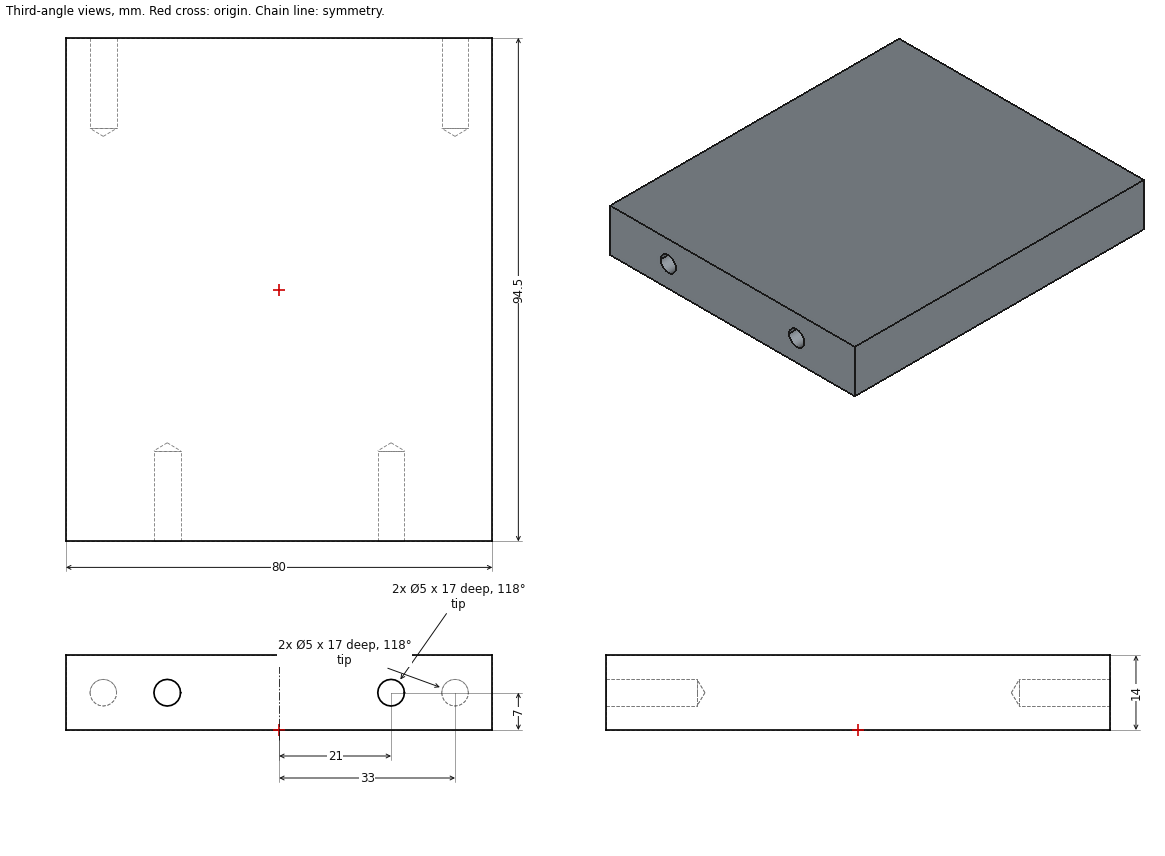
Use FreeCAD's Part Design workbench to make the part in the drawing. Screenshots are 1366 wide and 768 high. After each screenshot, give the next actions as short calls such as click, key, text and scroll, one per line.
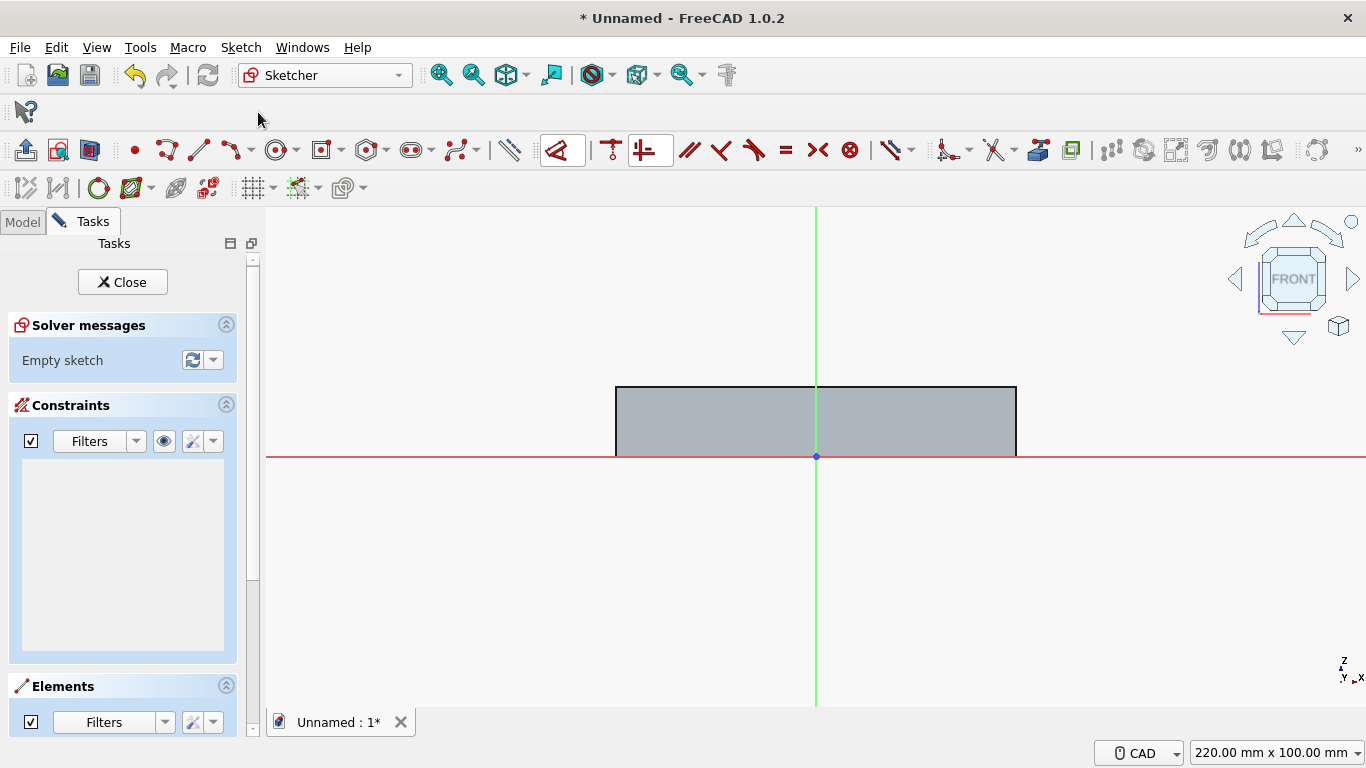
scroll(856, 419, up, 5)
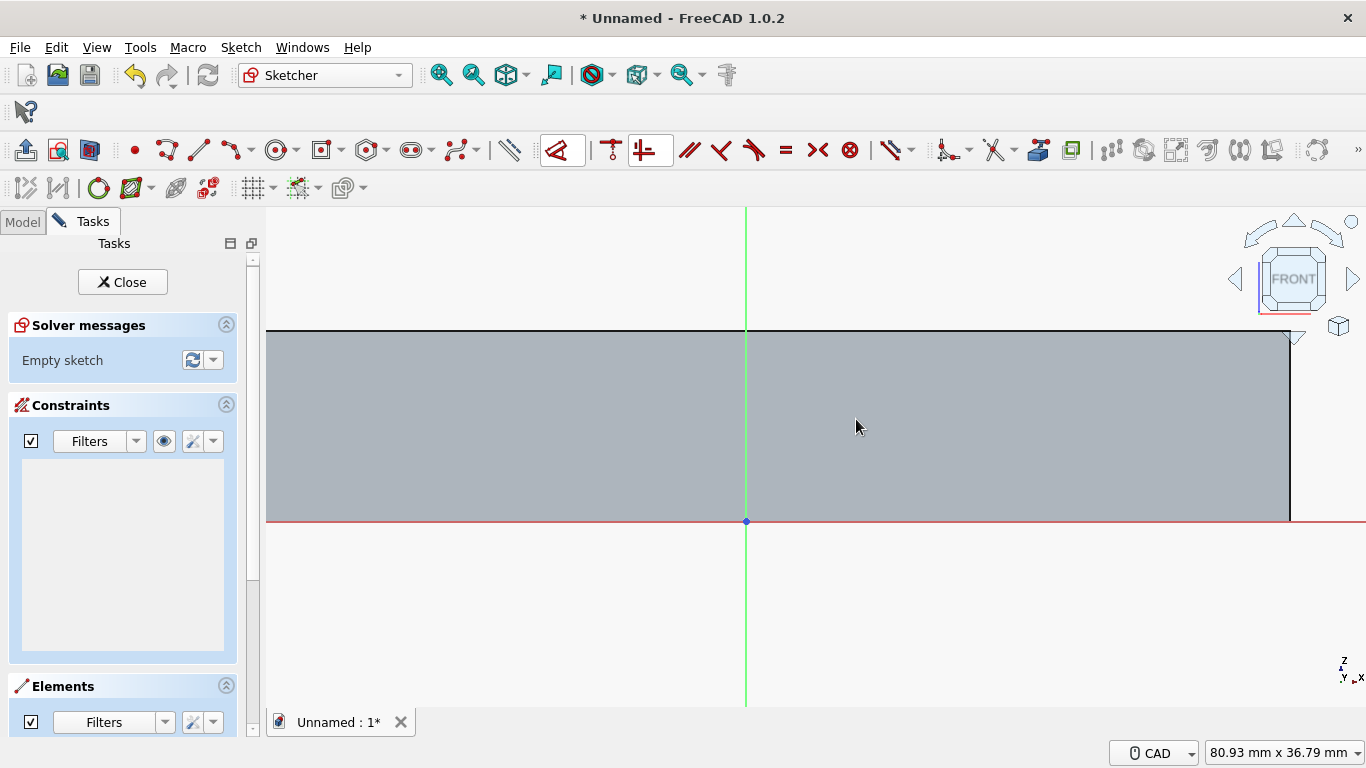
key(g)
key(c)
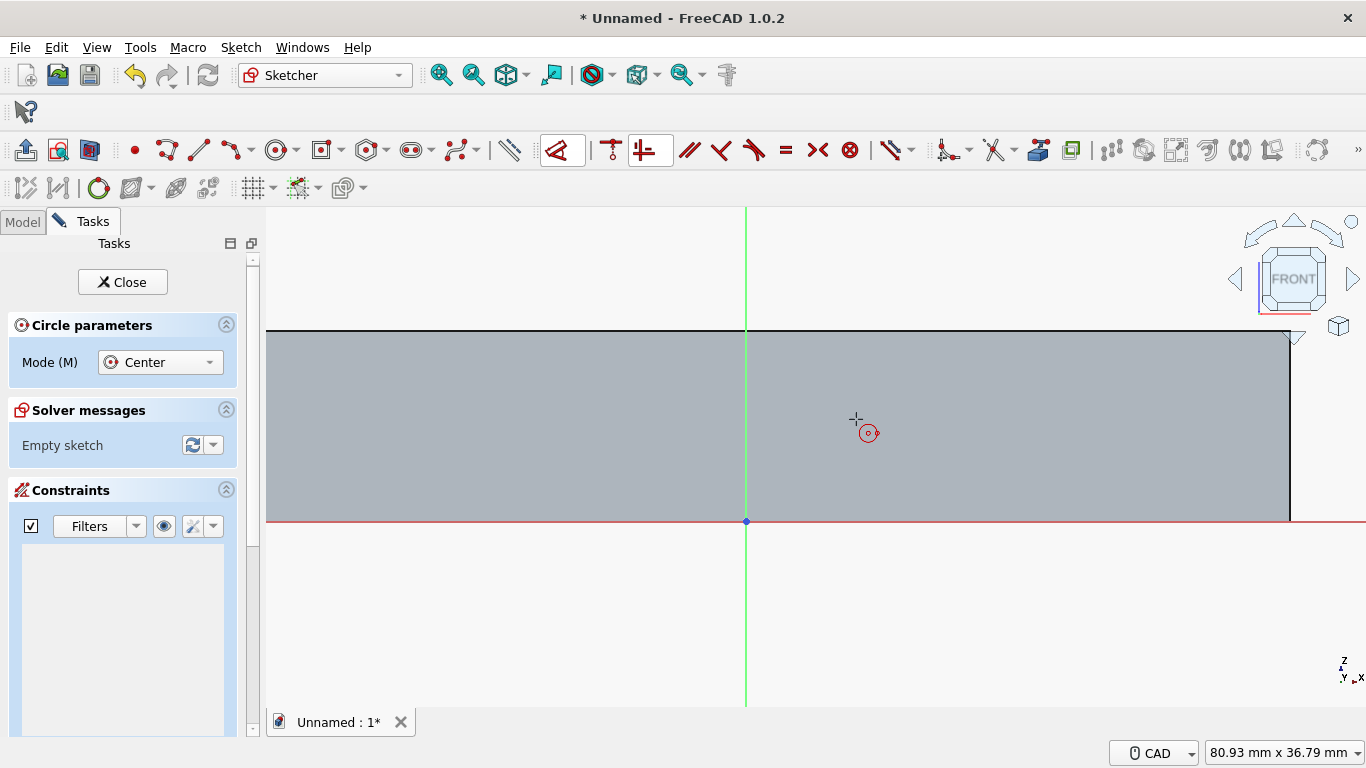
click(1032, 426)
click(1056, 402)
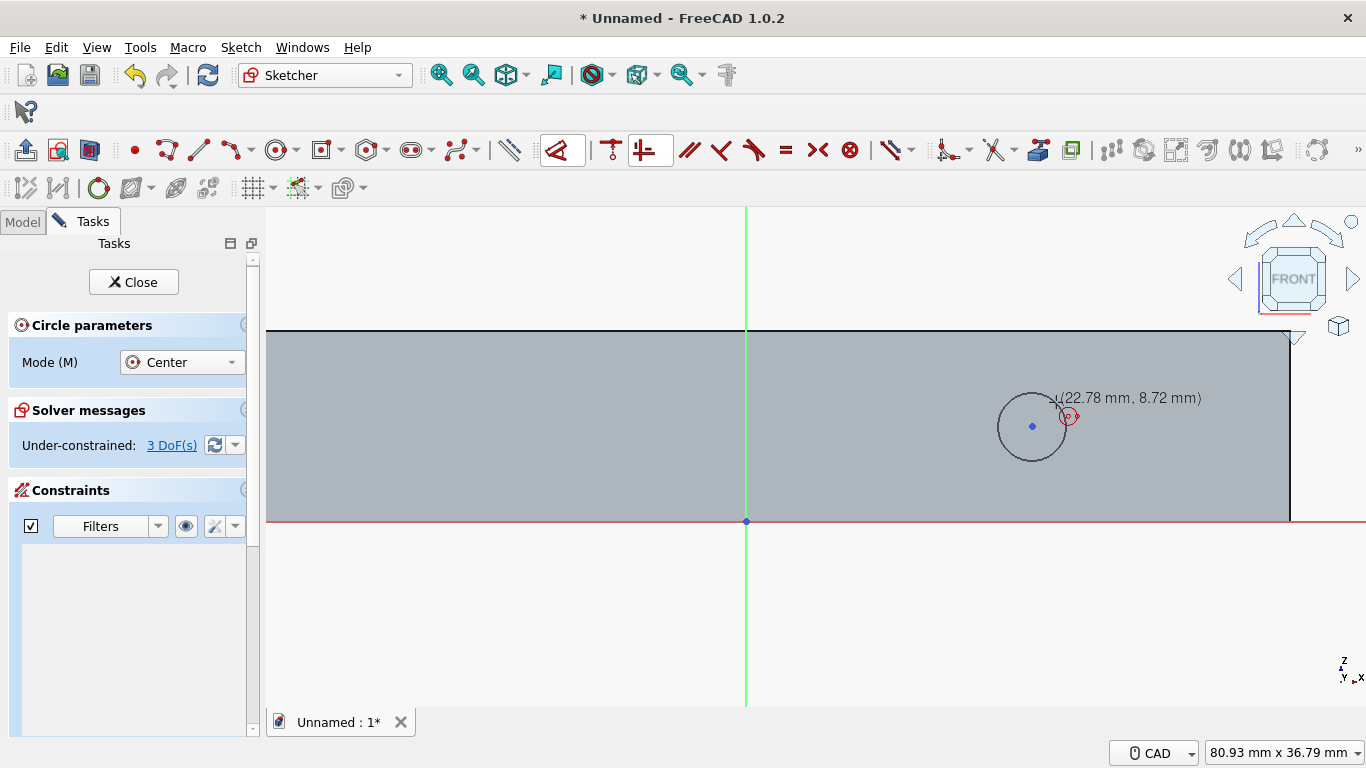
click(461, 426)
click(485, 402)
key(Escape)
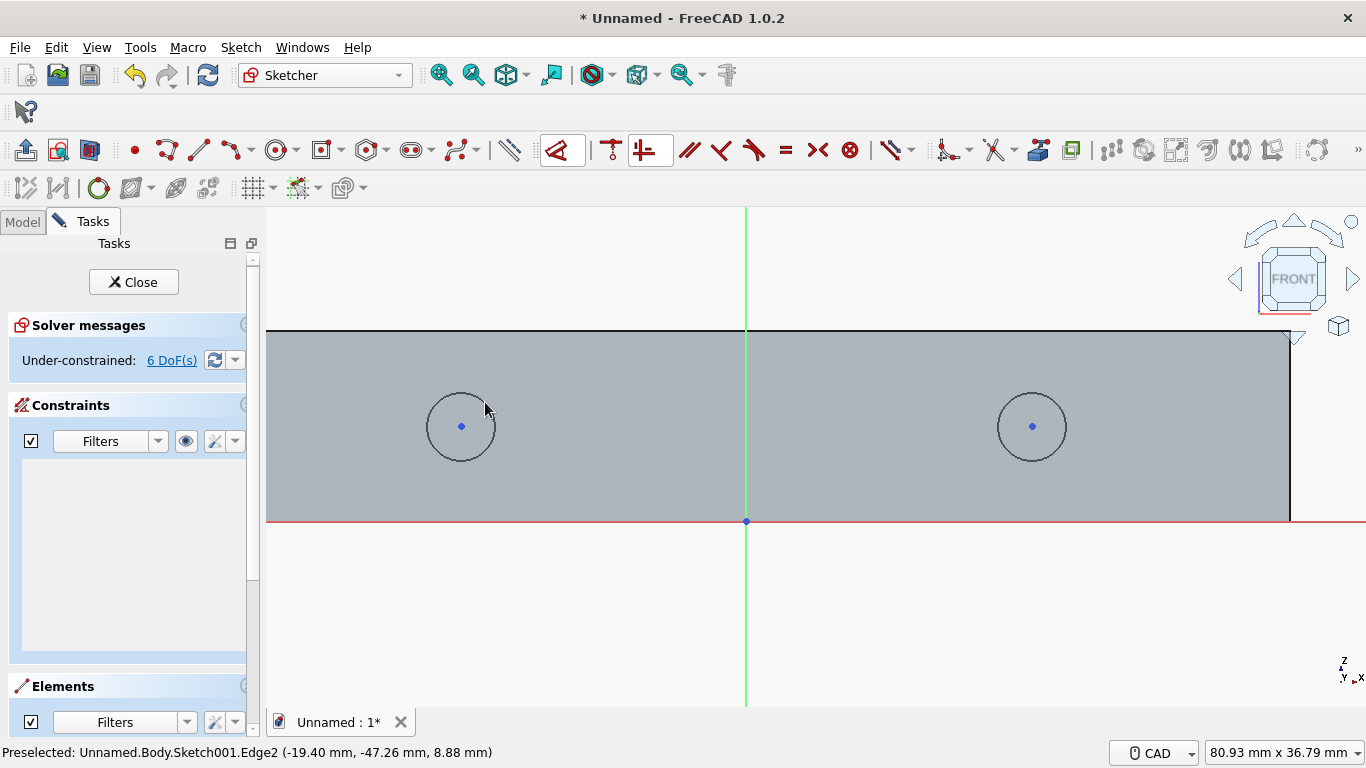
click(1056, 403)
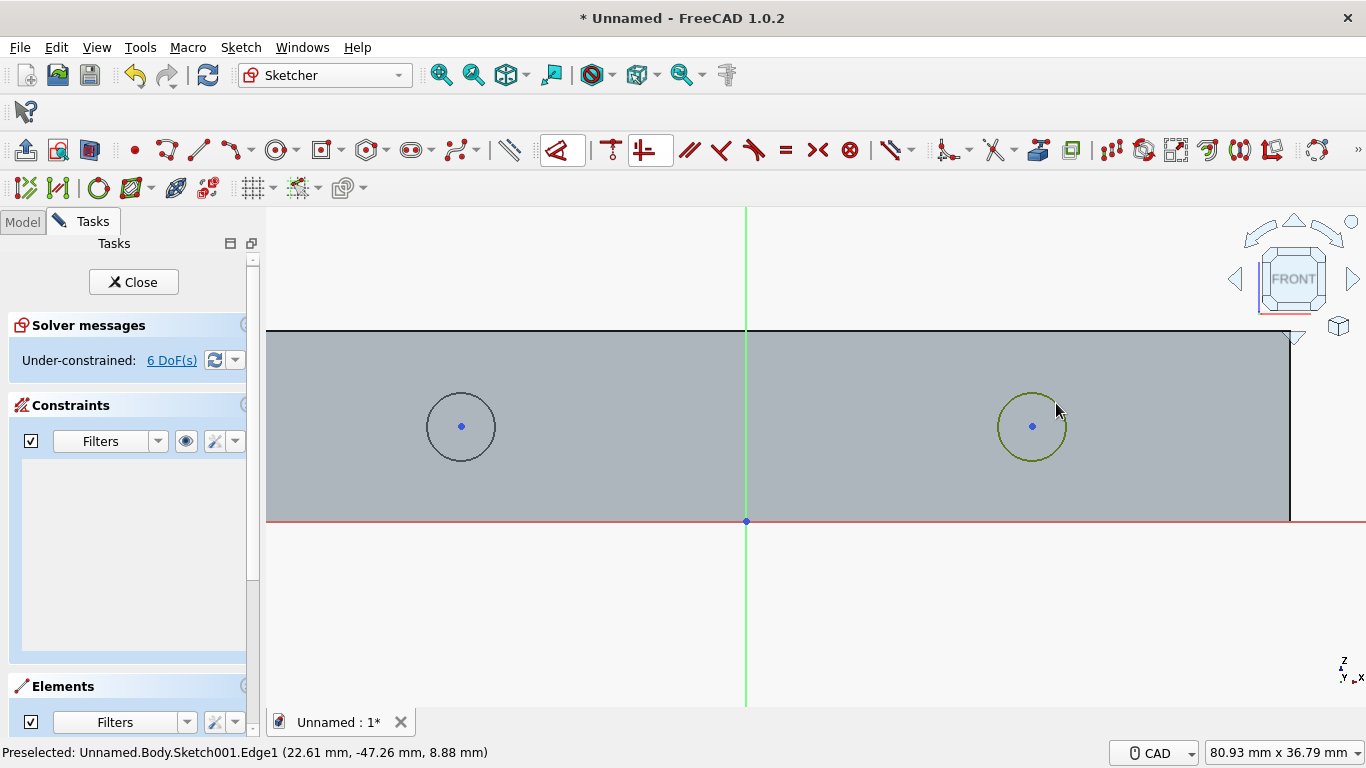
click(485, 403)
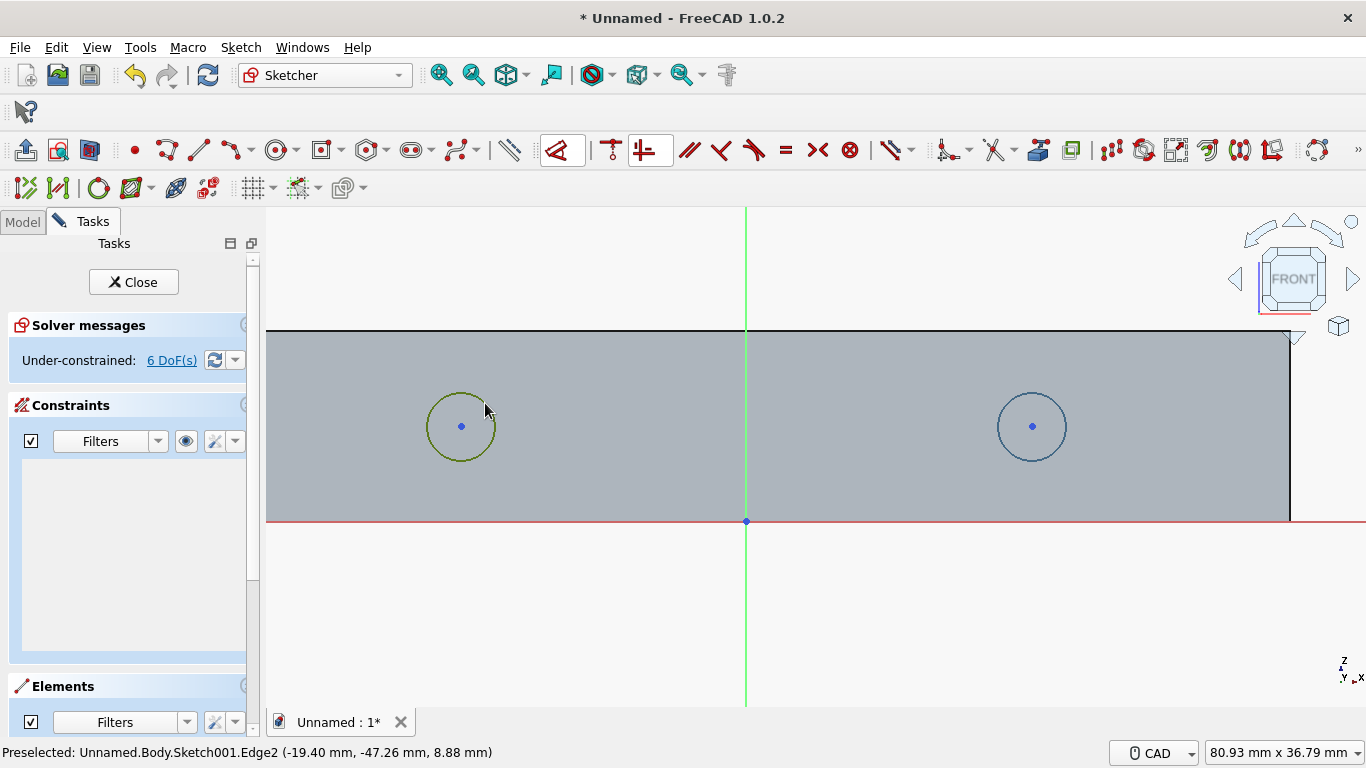
key(e)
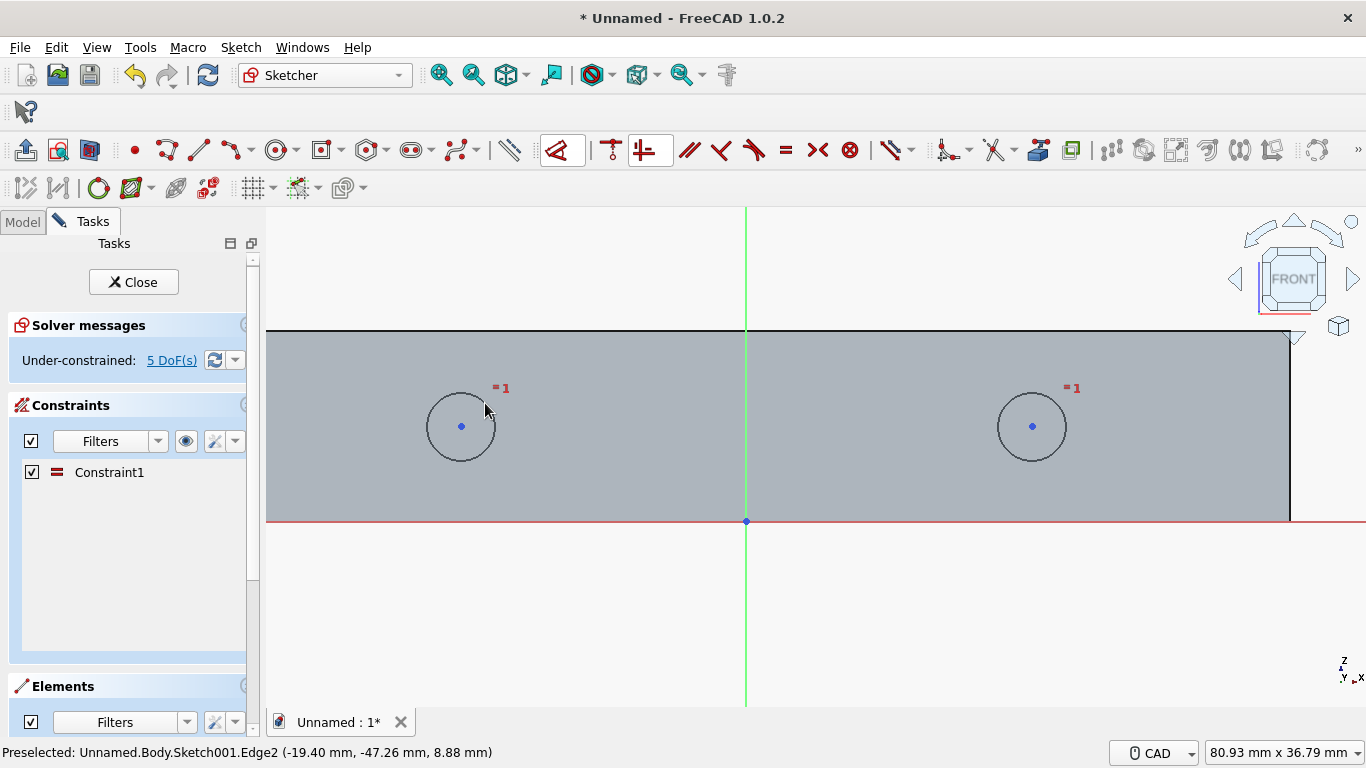
click(1032, 427)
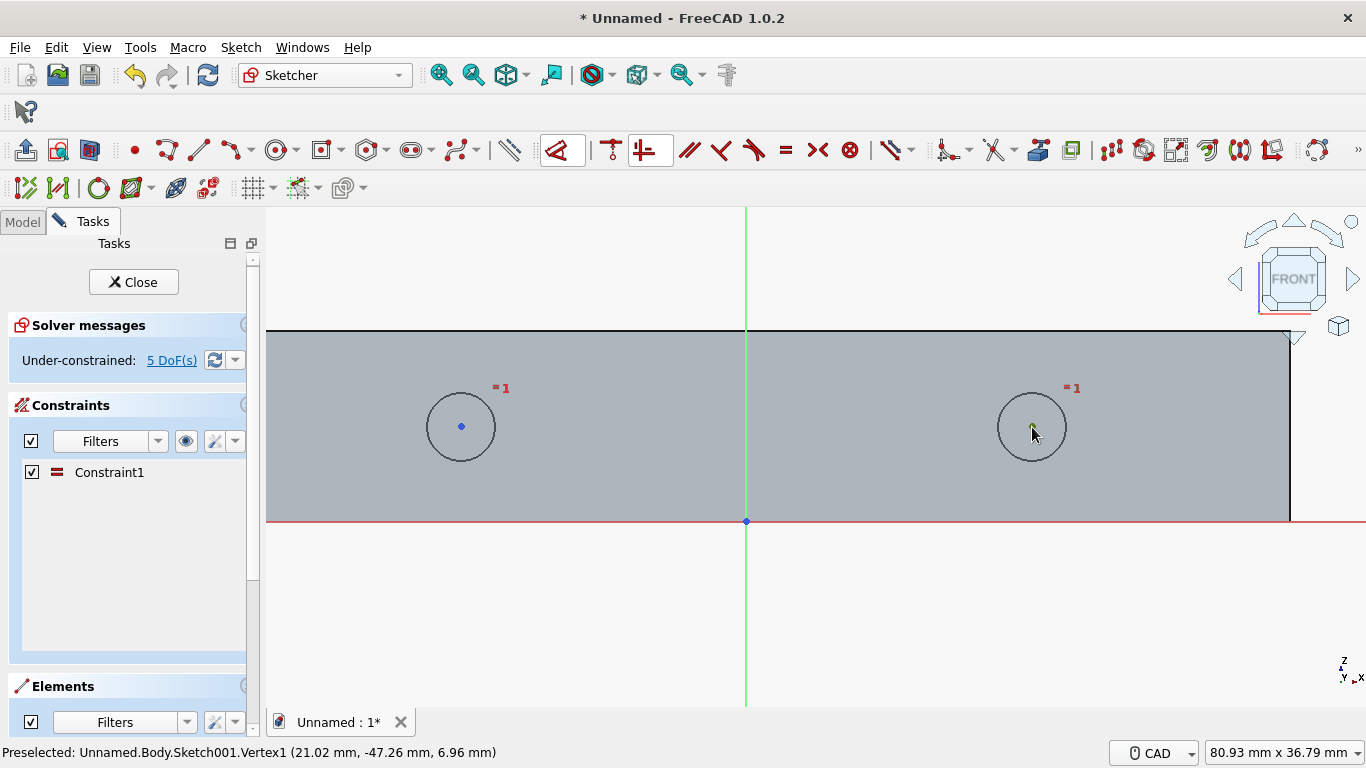
click(461, 427)